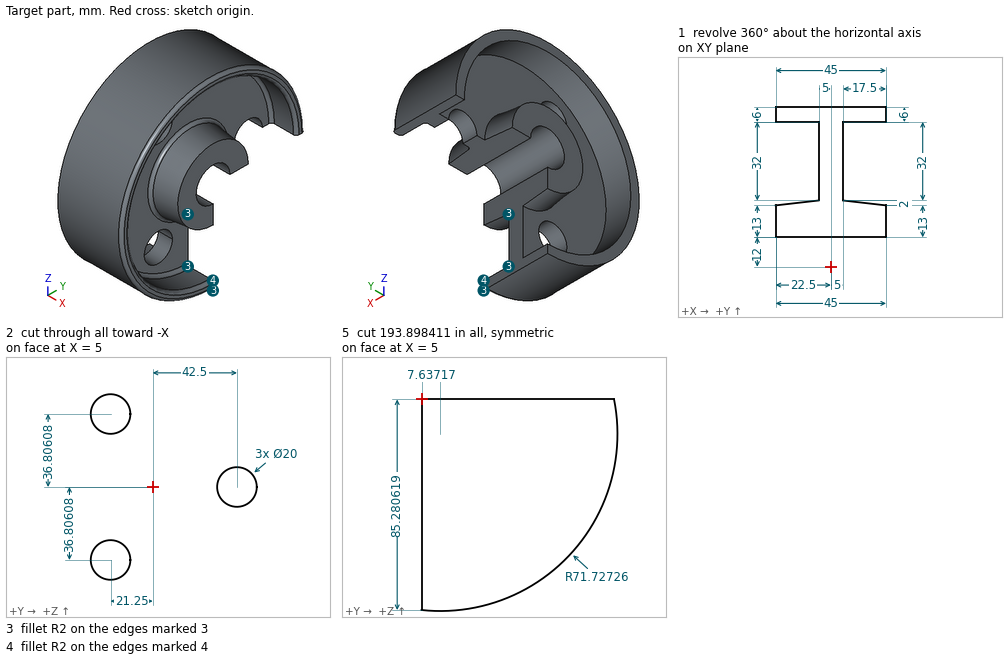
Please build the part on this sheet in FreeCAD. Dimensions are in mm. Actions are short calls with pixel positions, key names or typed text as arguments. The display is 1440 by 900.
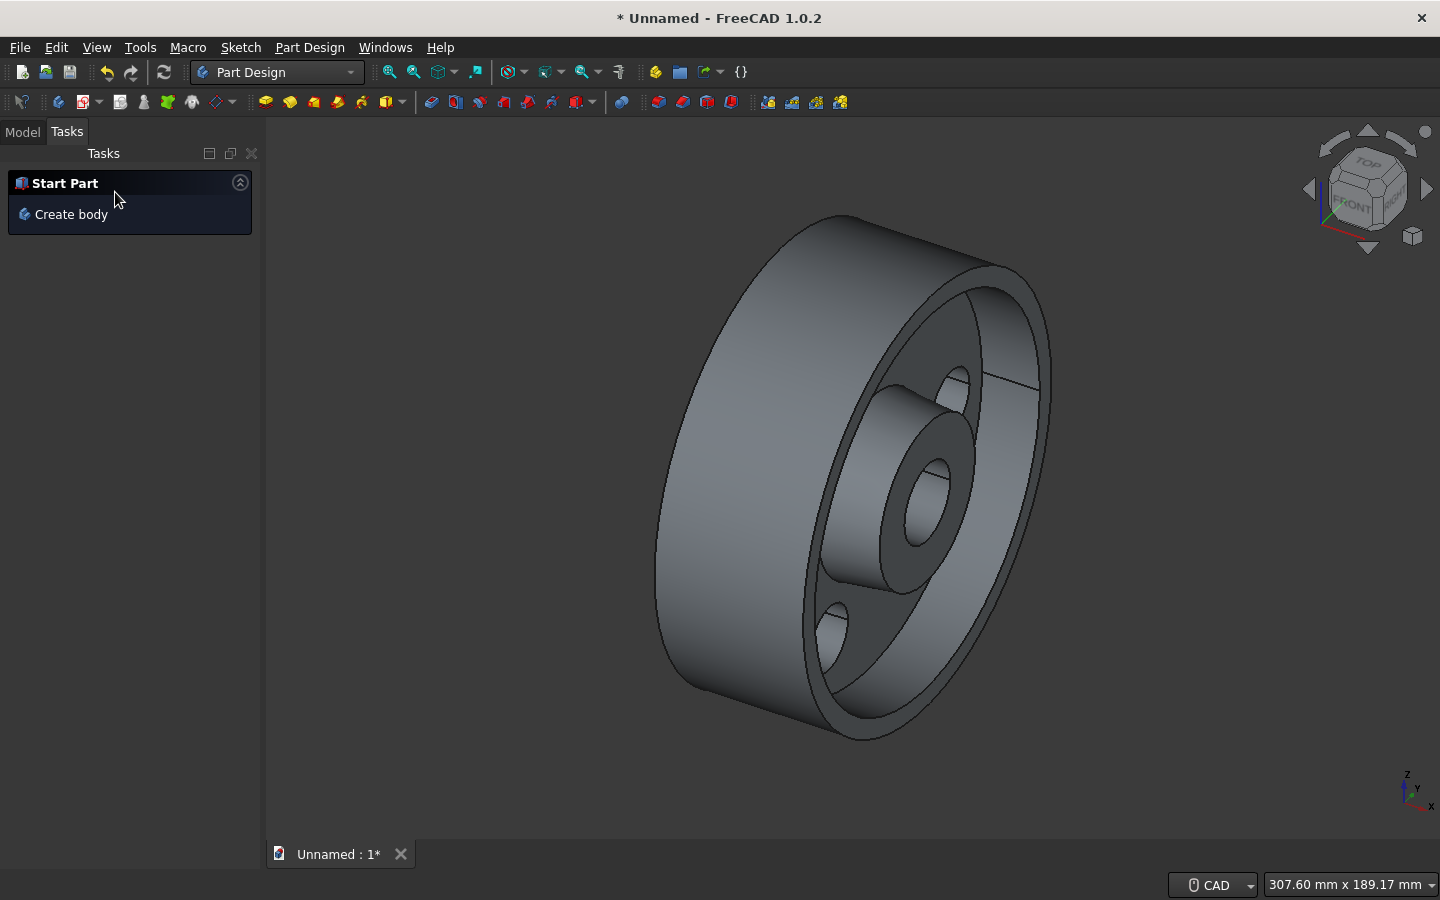
click(803, 625)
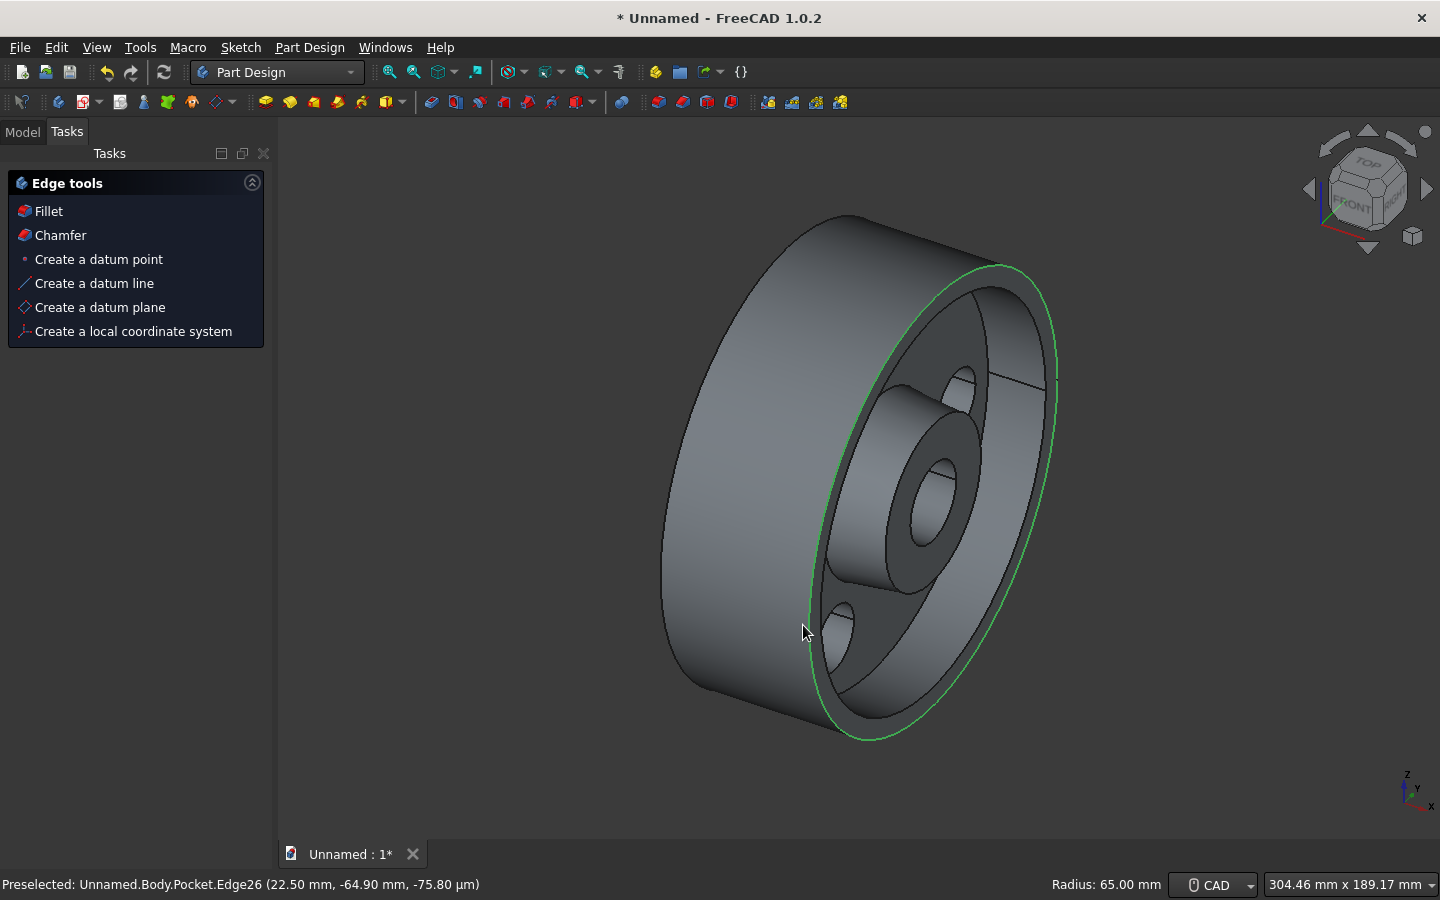
key(0)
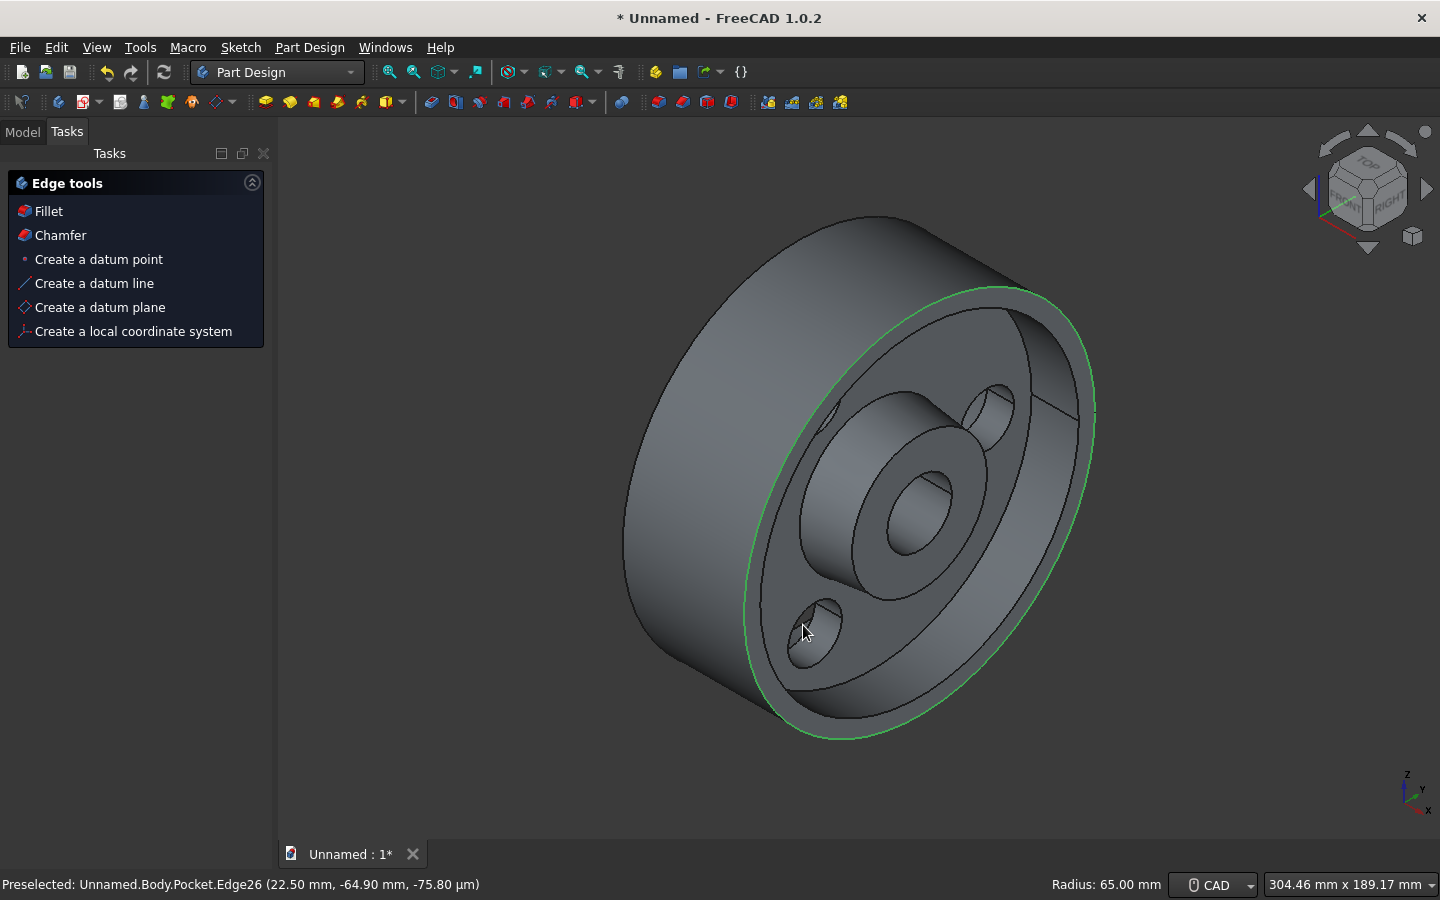
key(2)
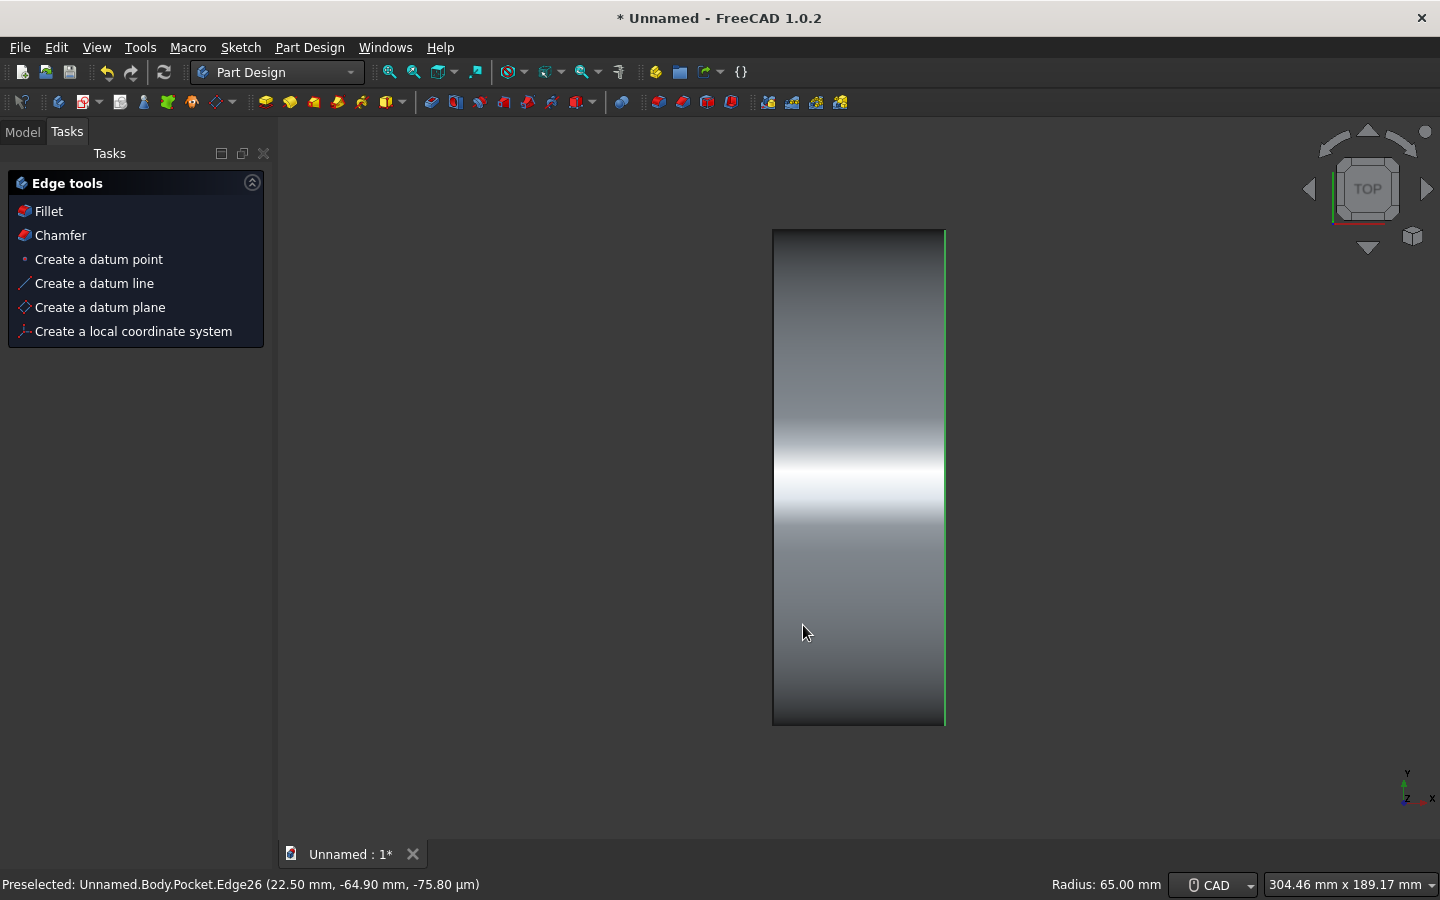
key(1)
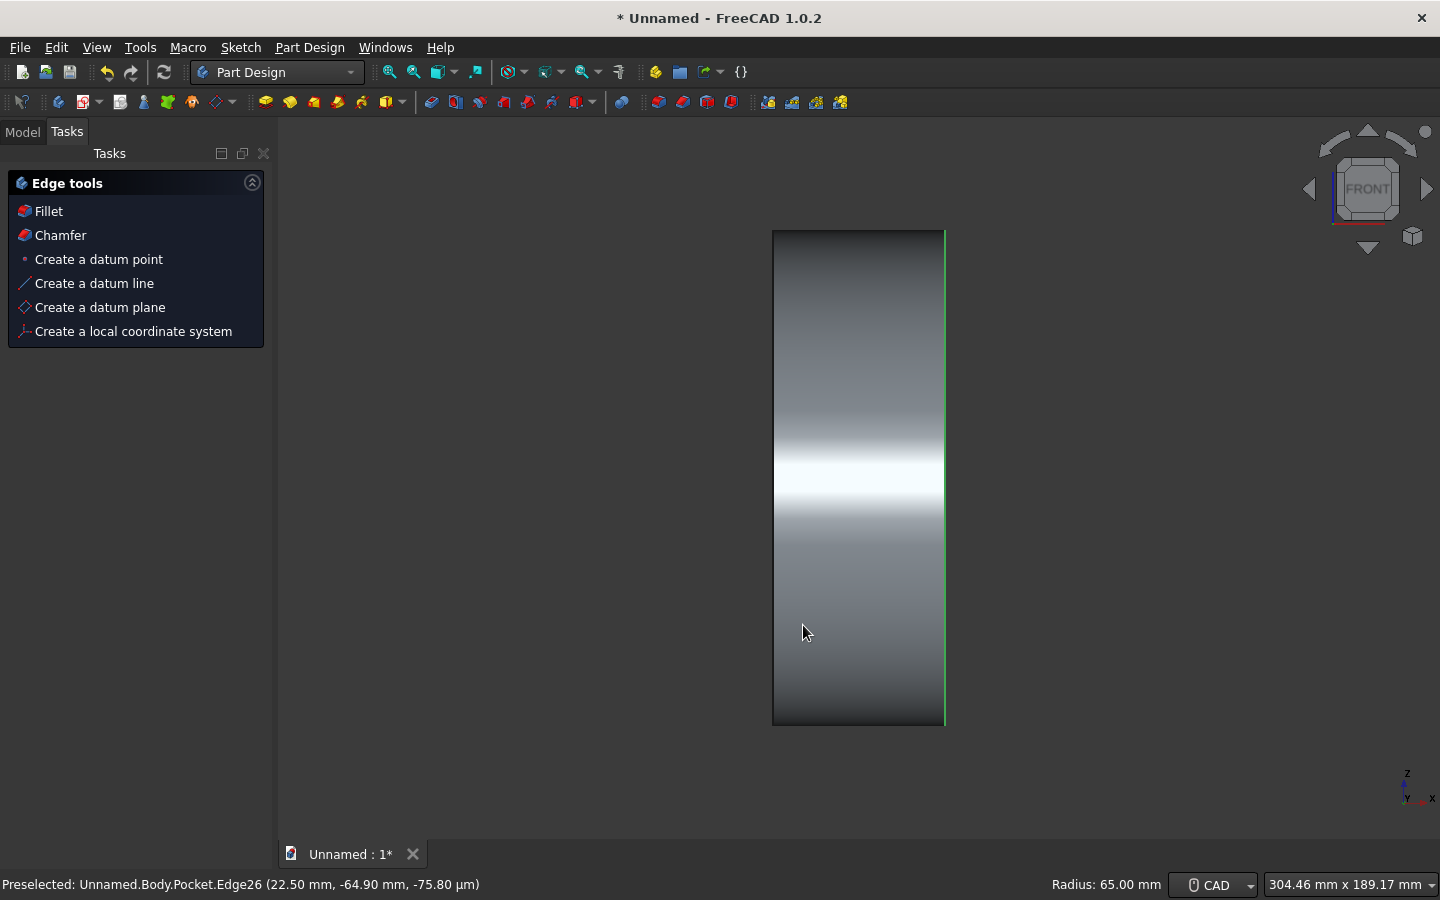
key(3)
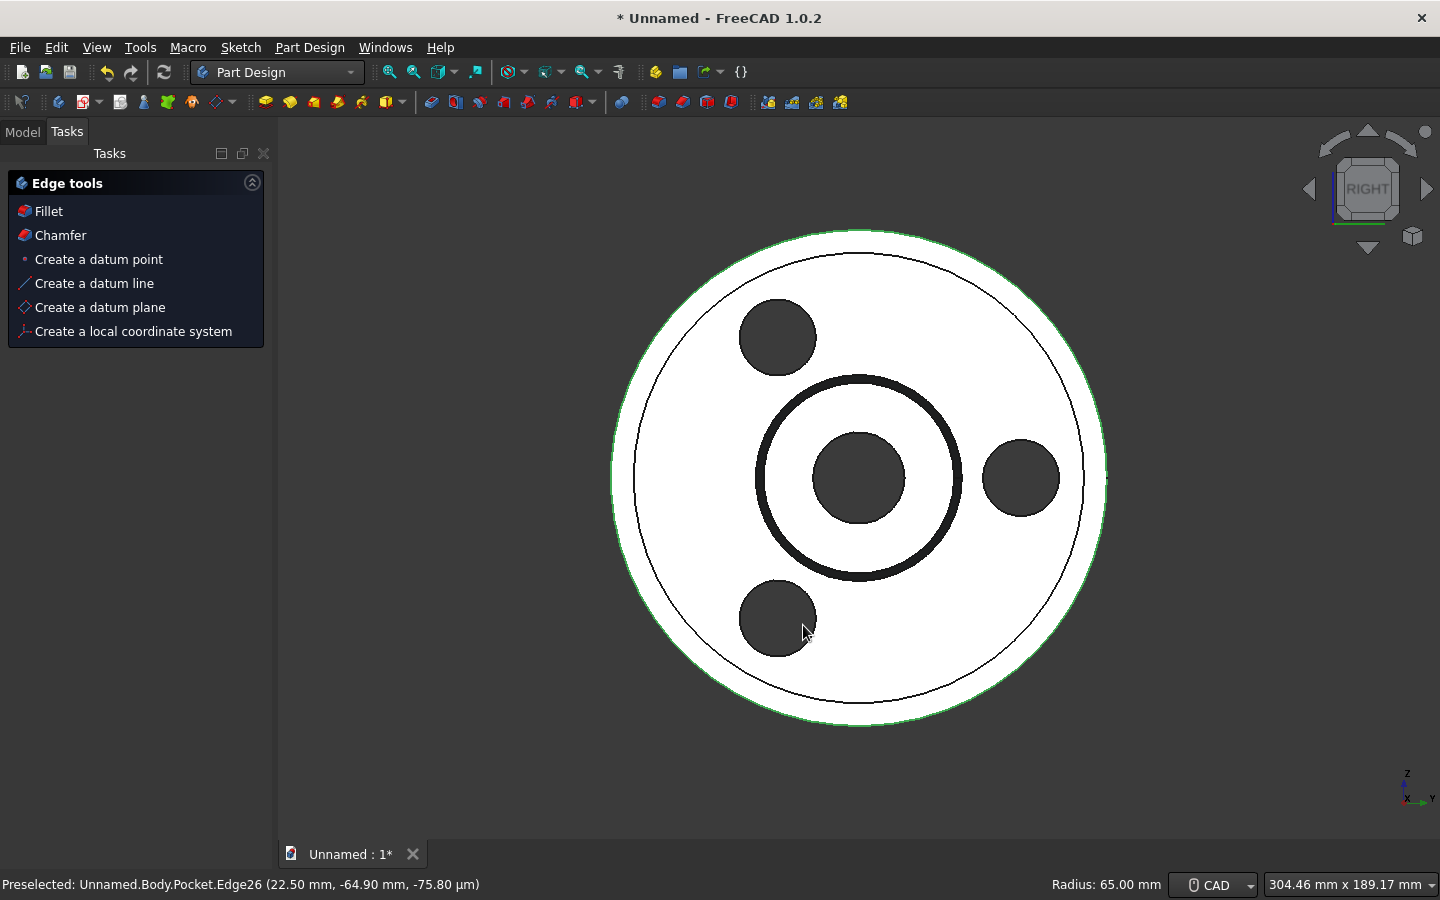
key(5)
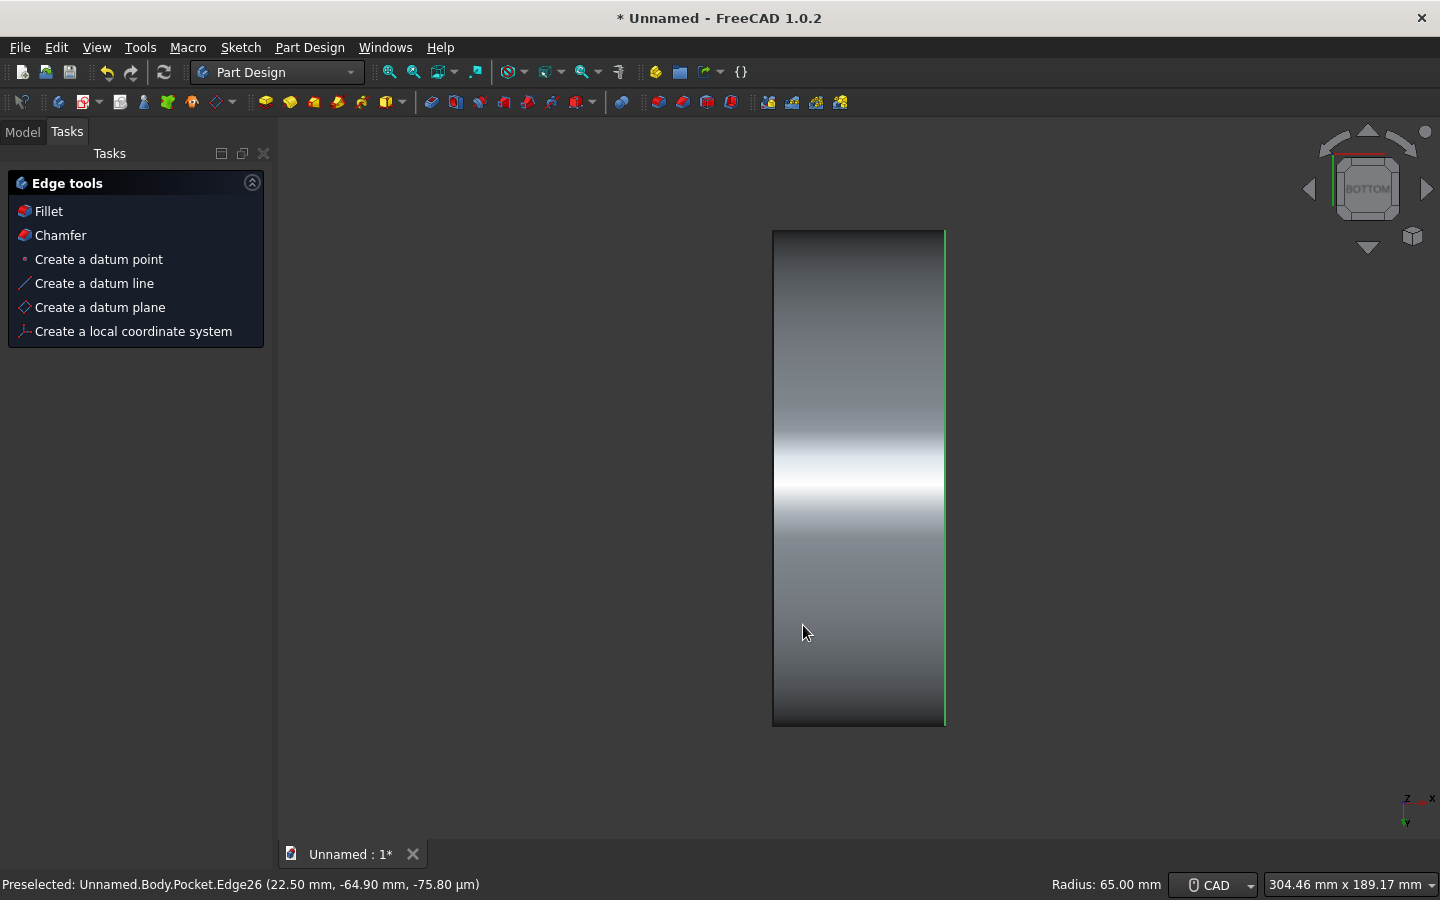
key(4)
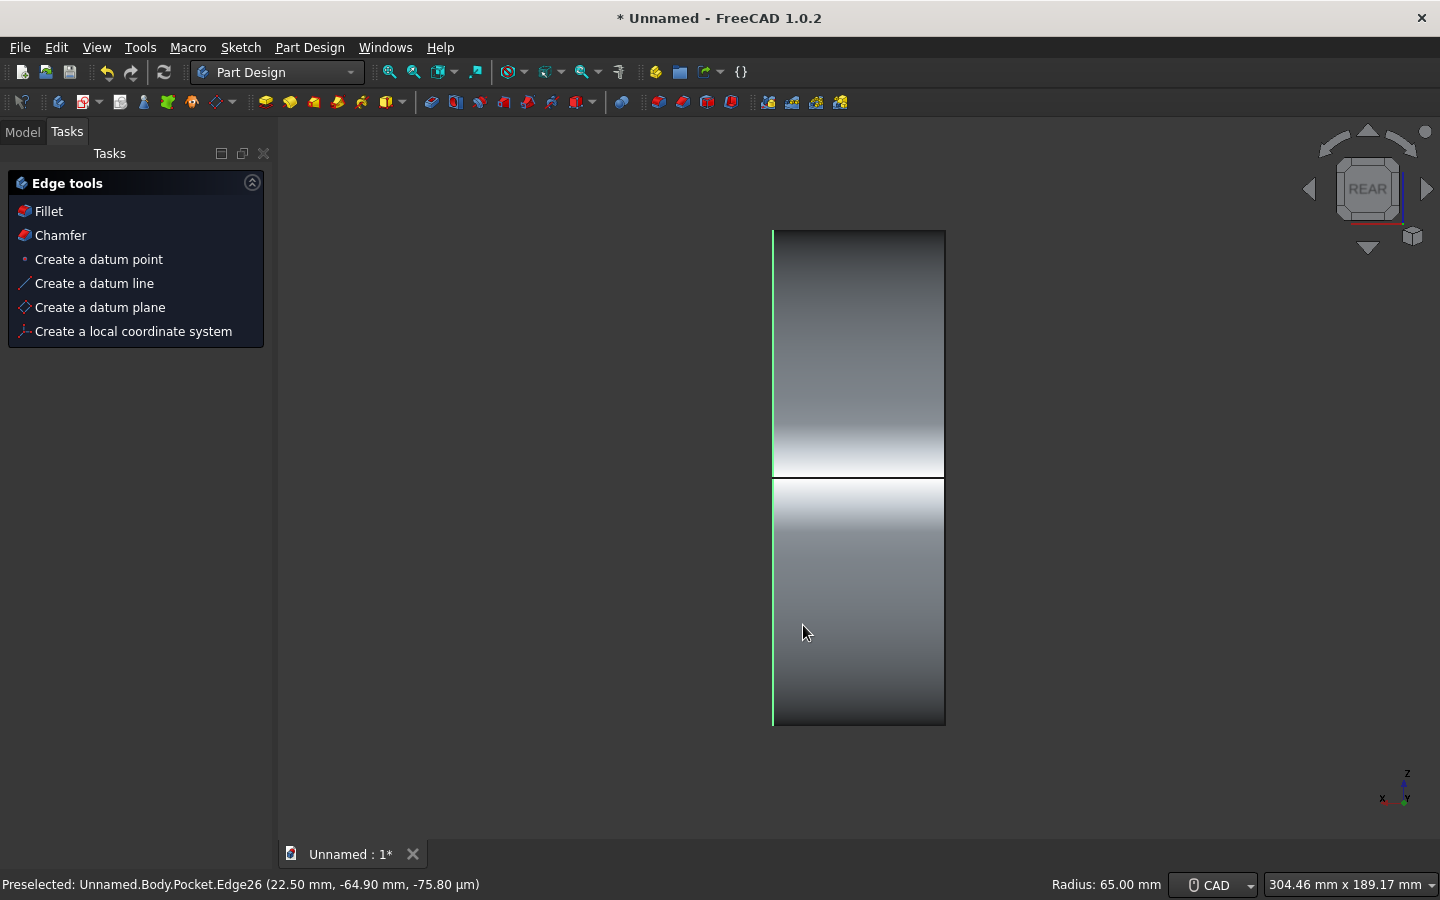
key(6)